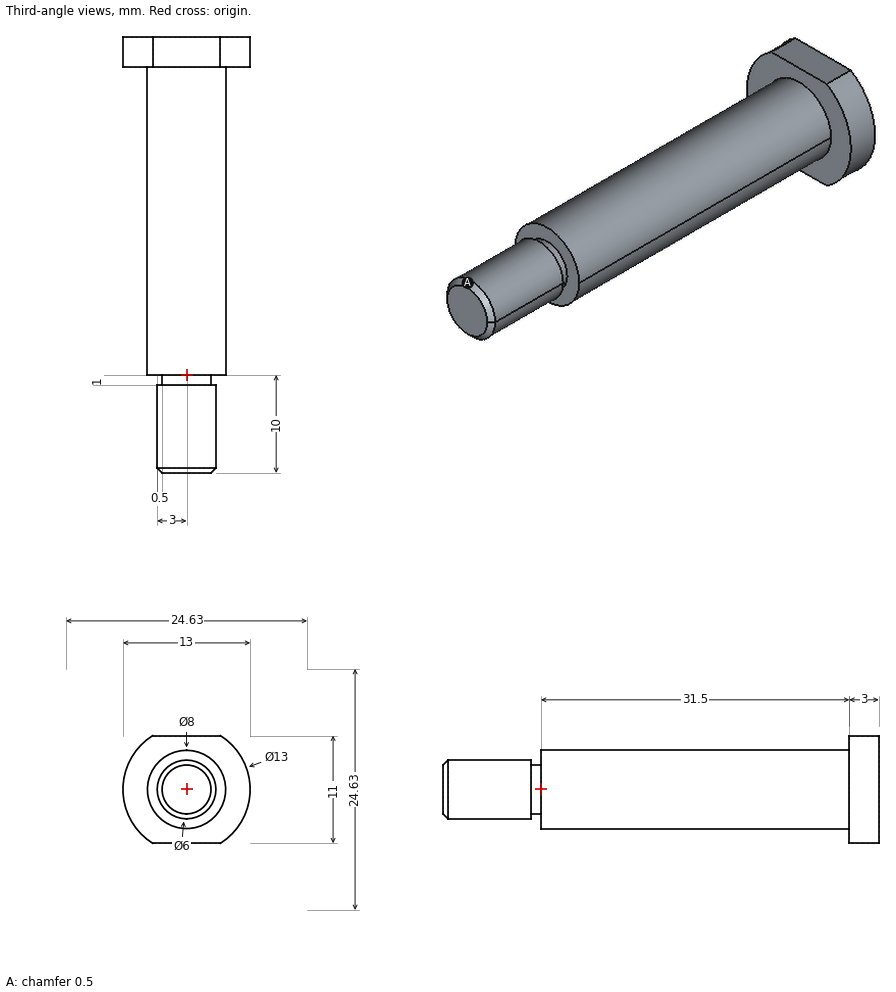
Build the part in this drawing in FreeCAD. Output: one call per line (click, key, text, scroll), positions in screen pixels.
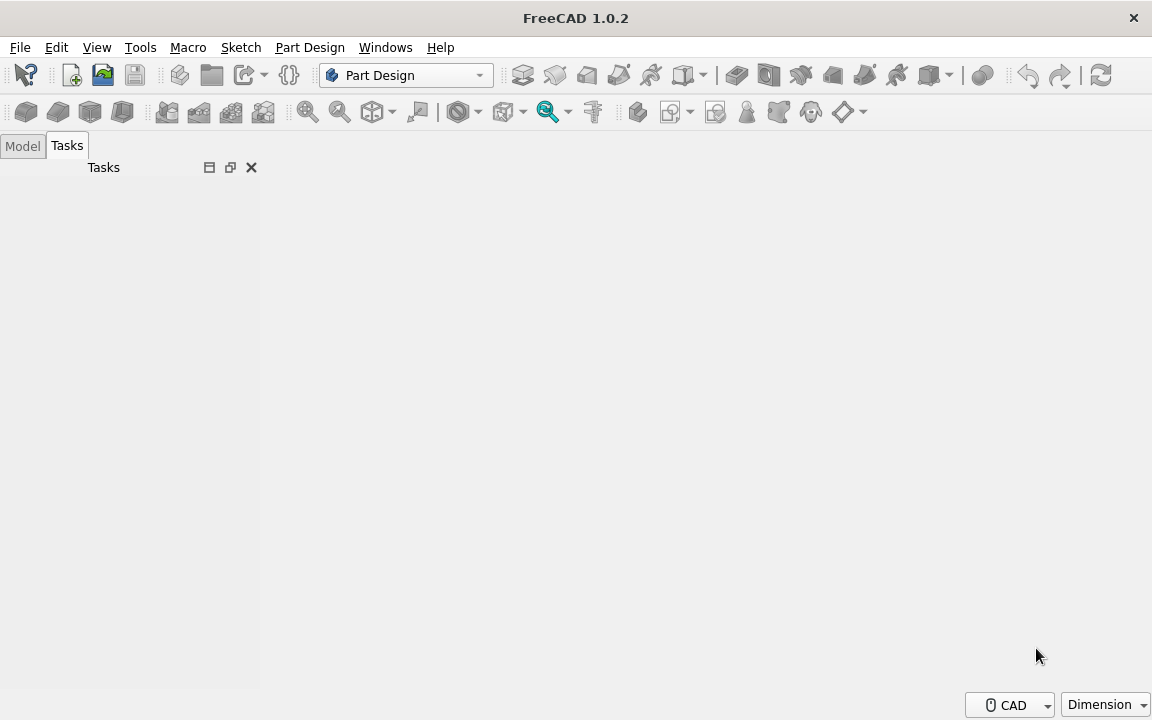
click(72, 76)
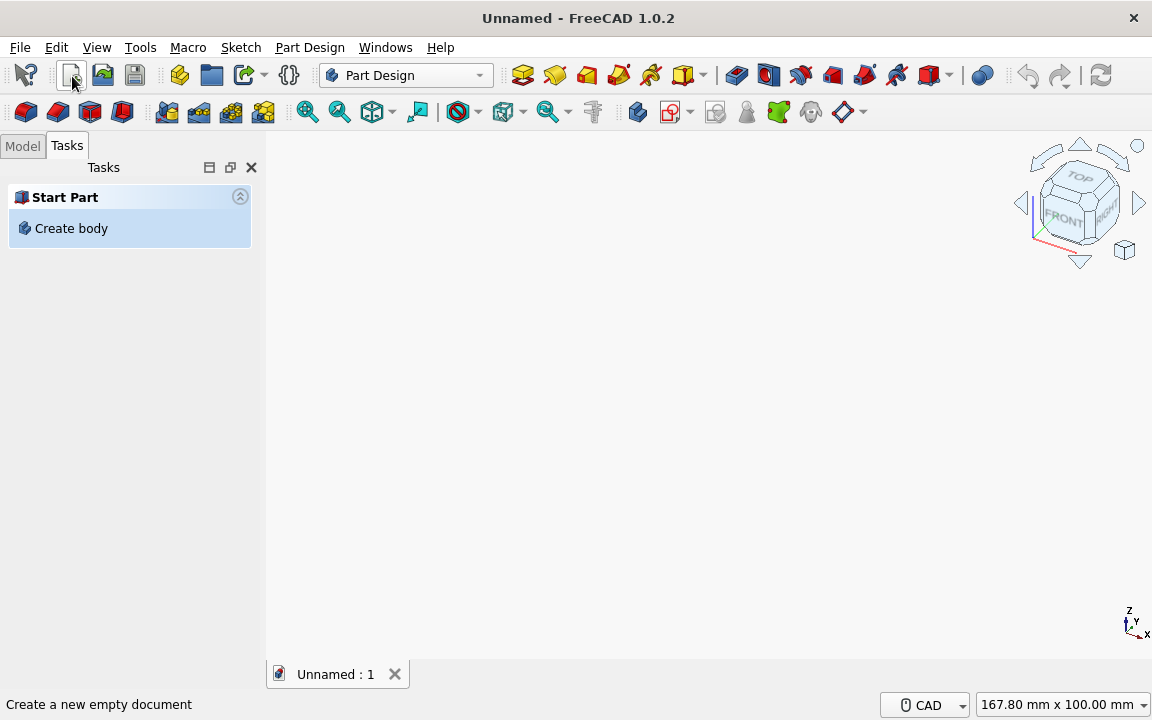
click(670, 112)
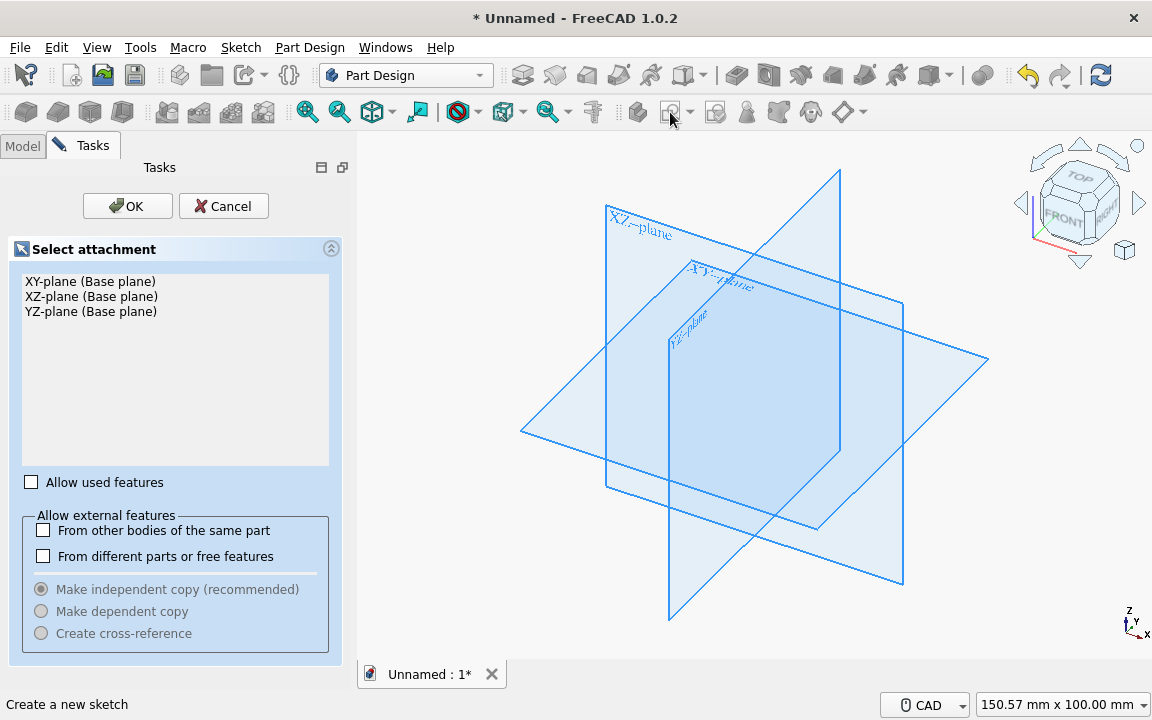
click(82, 296)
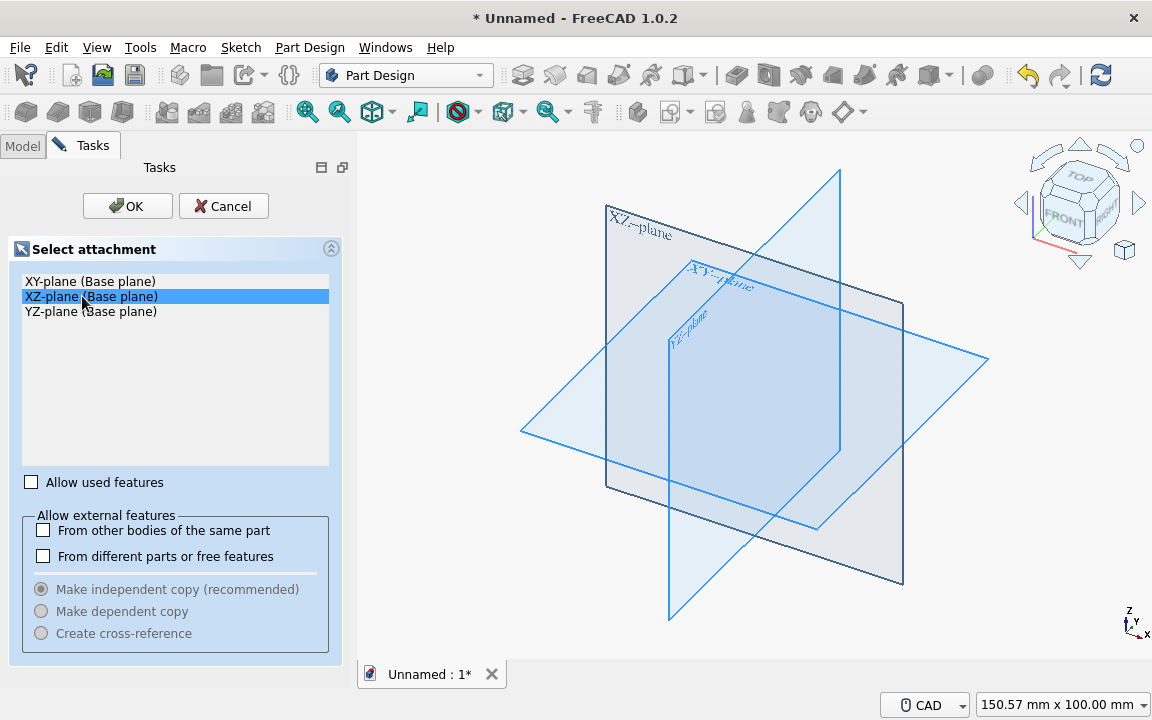
click(128, 206)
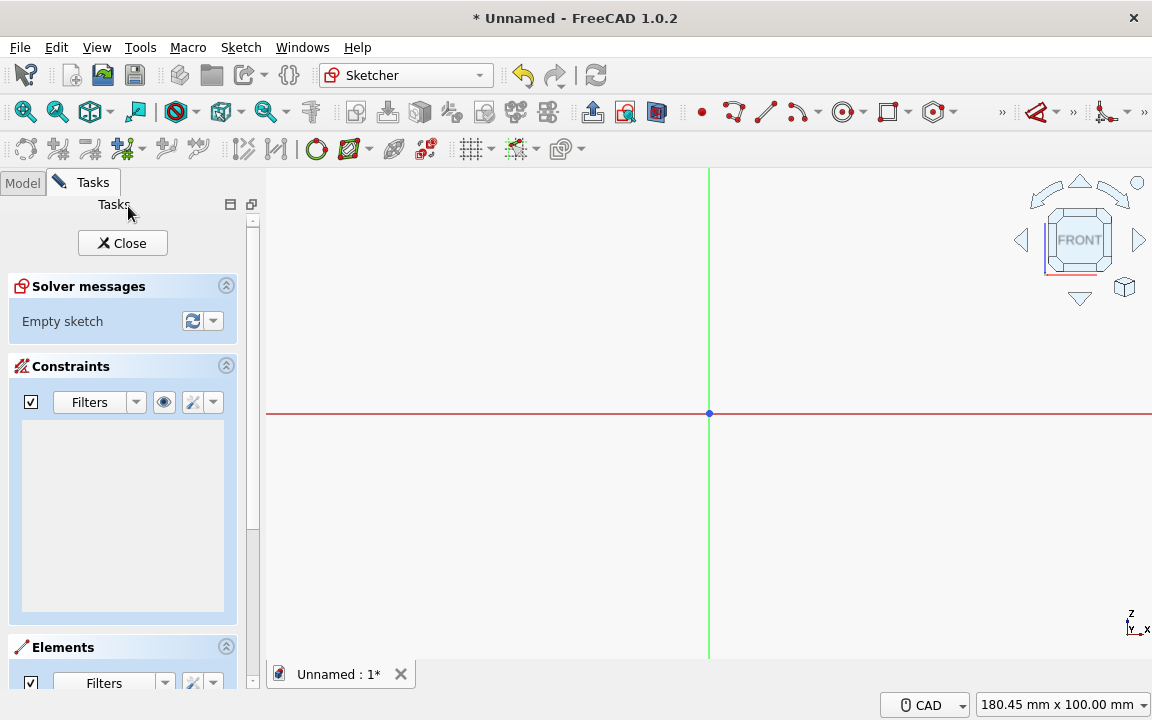
scroll(720, 414, up, 10)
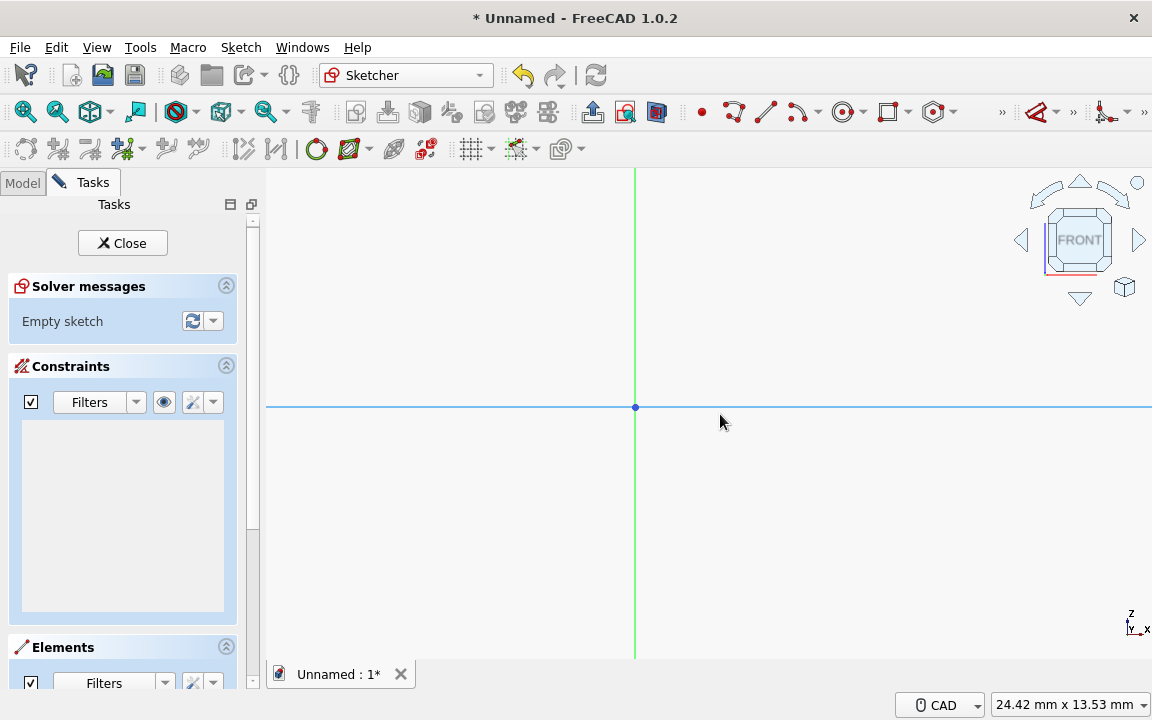
key(g)
key(c)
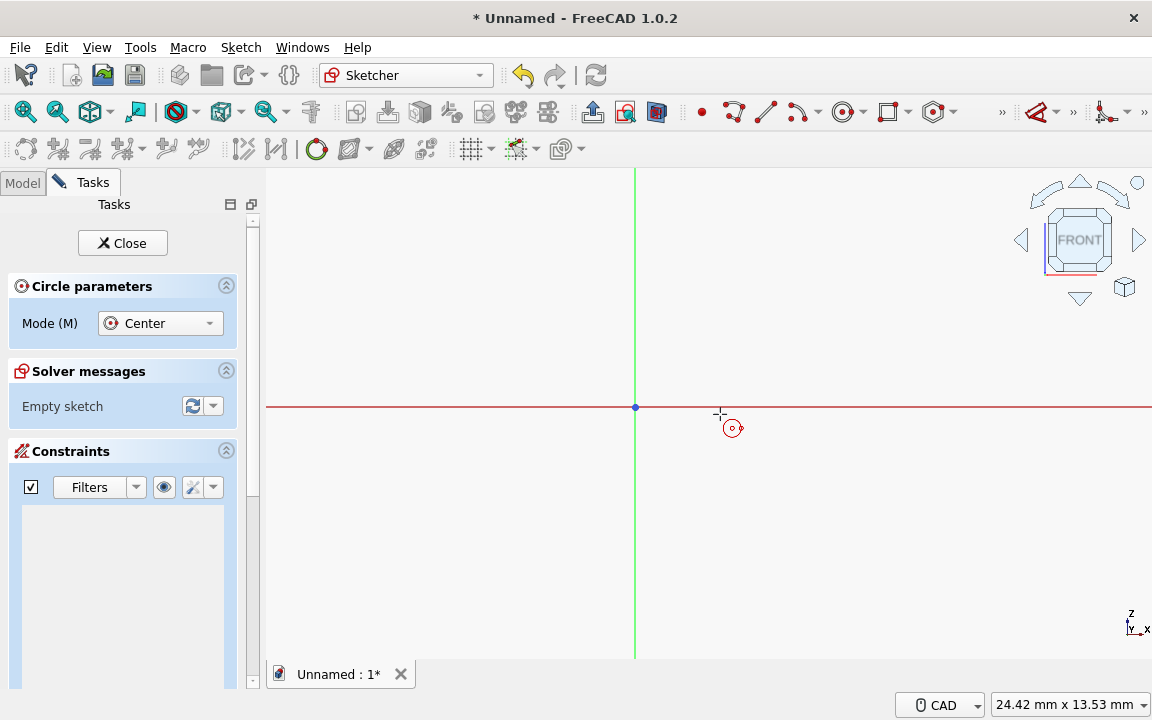
click(635, 407)
move(738, 304)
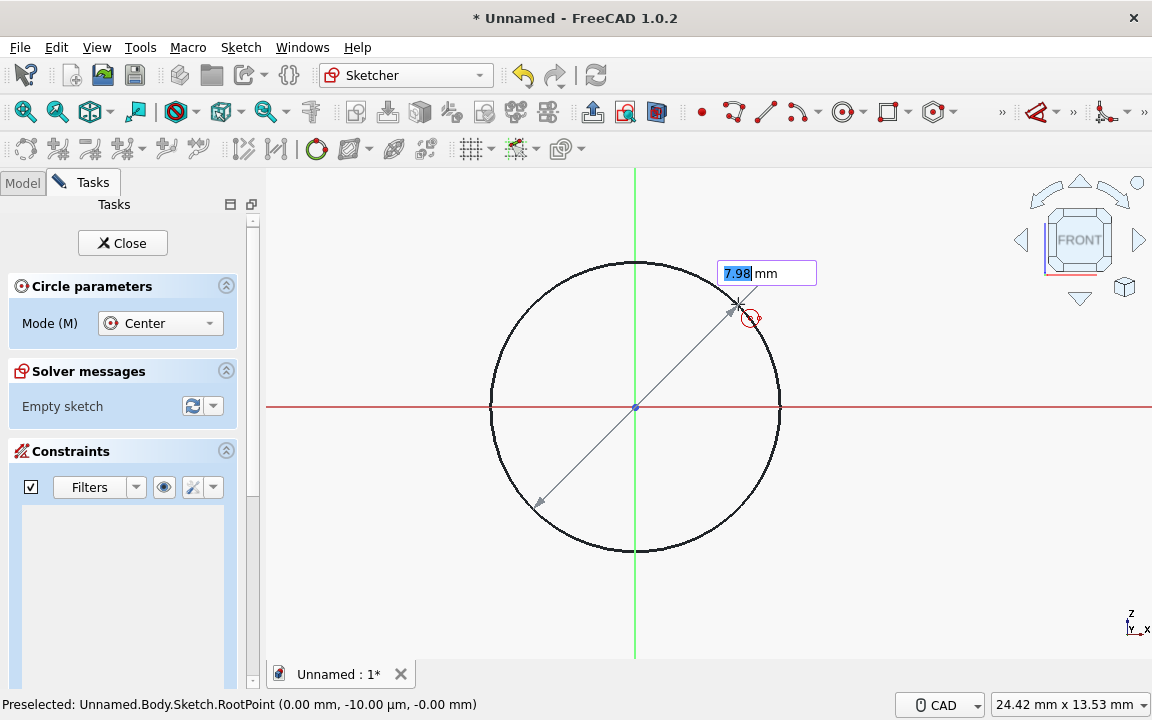
text(8)
key(Return)
key(Escape)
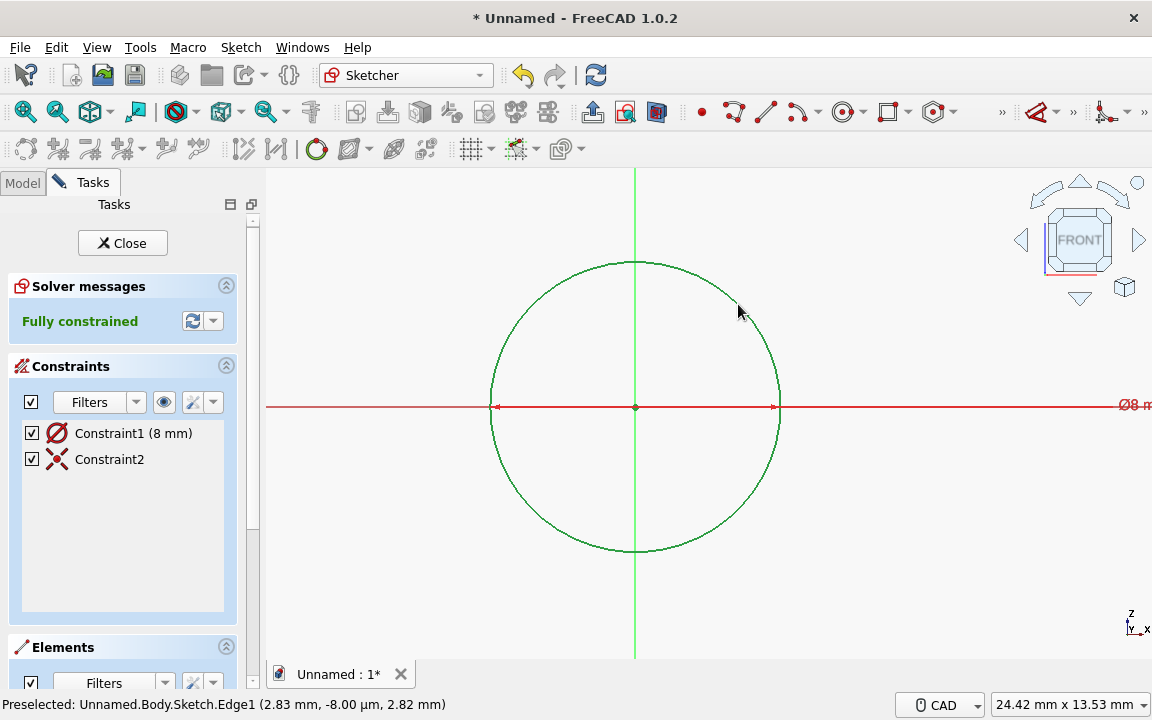
click(123, 243)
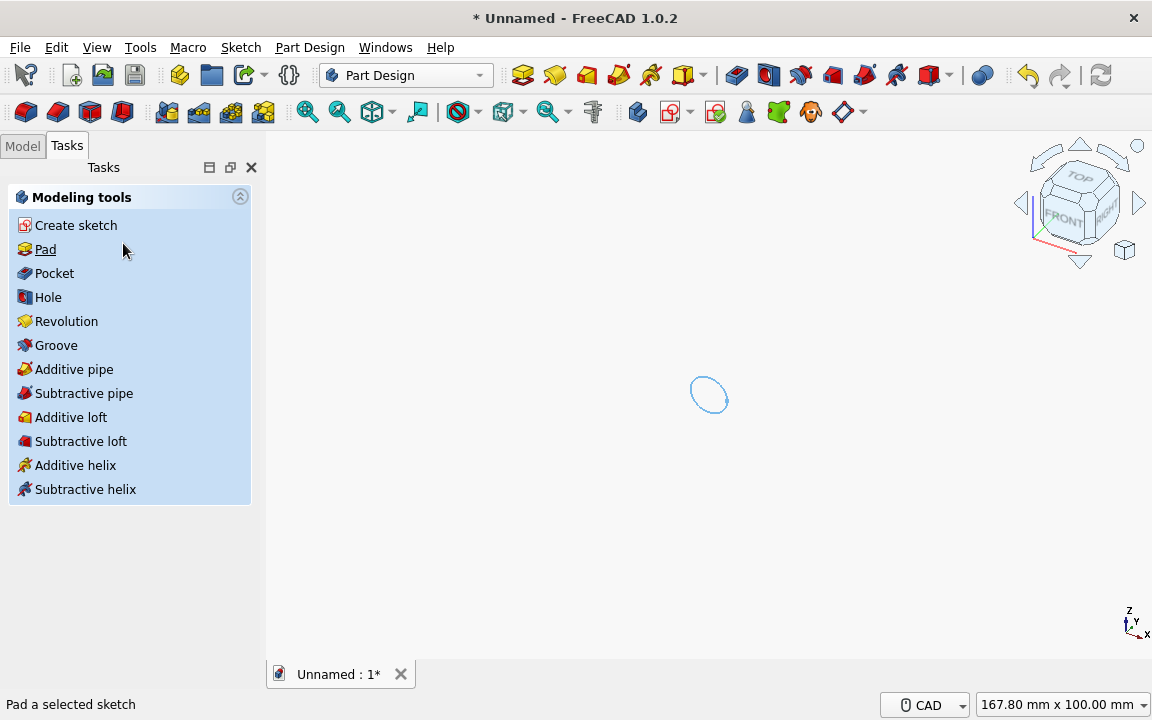
click(524, 76)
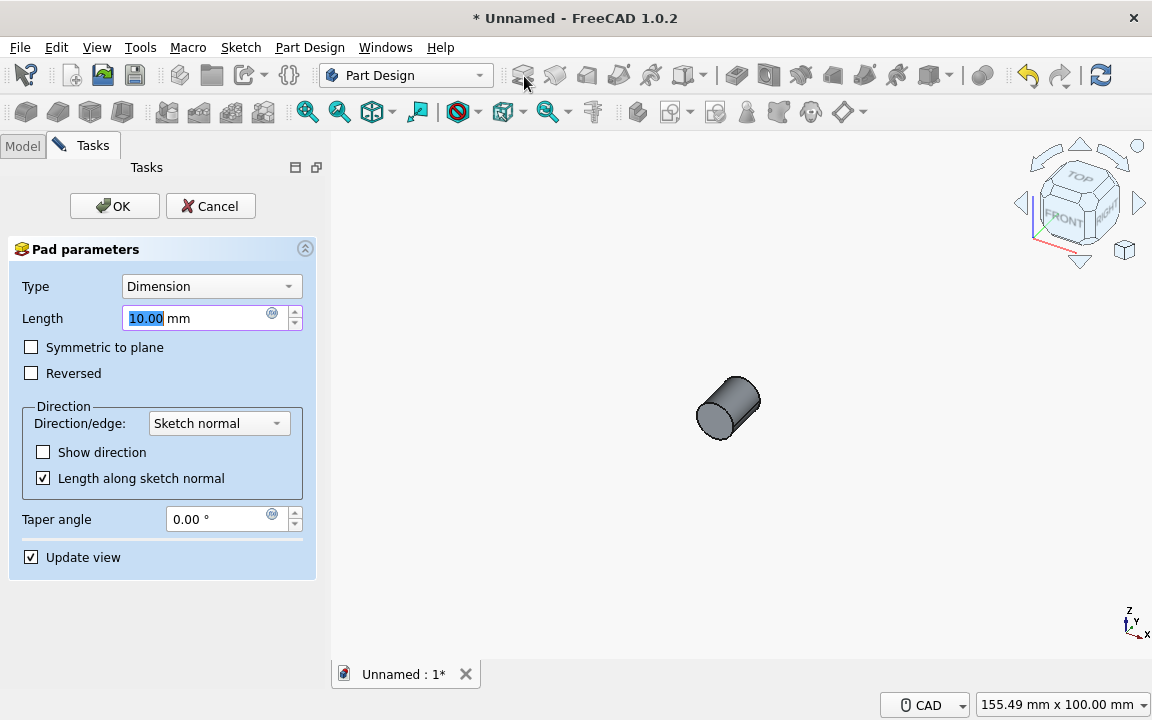
text(31.5)
key(Tab)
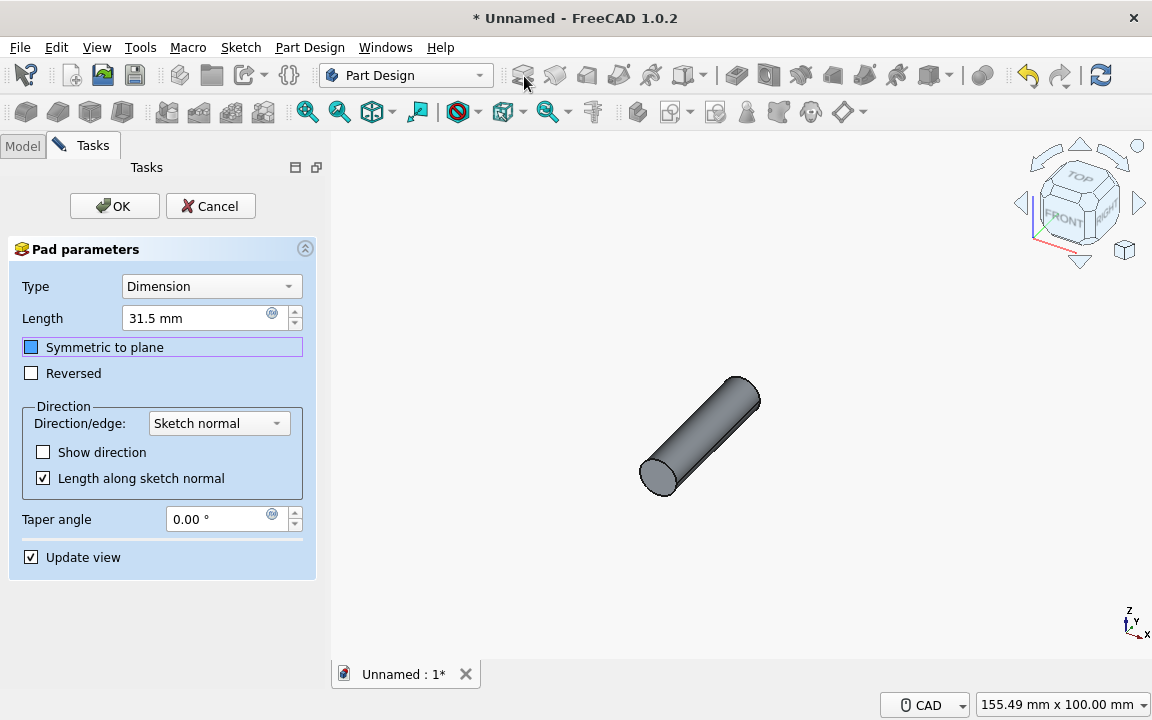
click(30, 373)